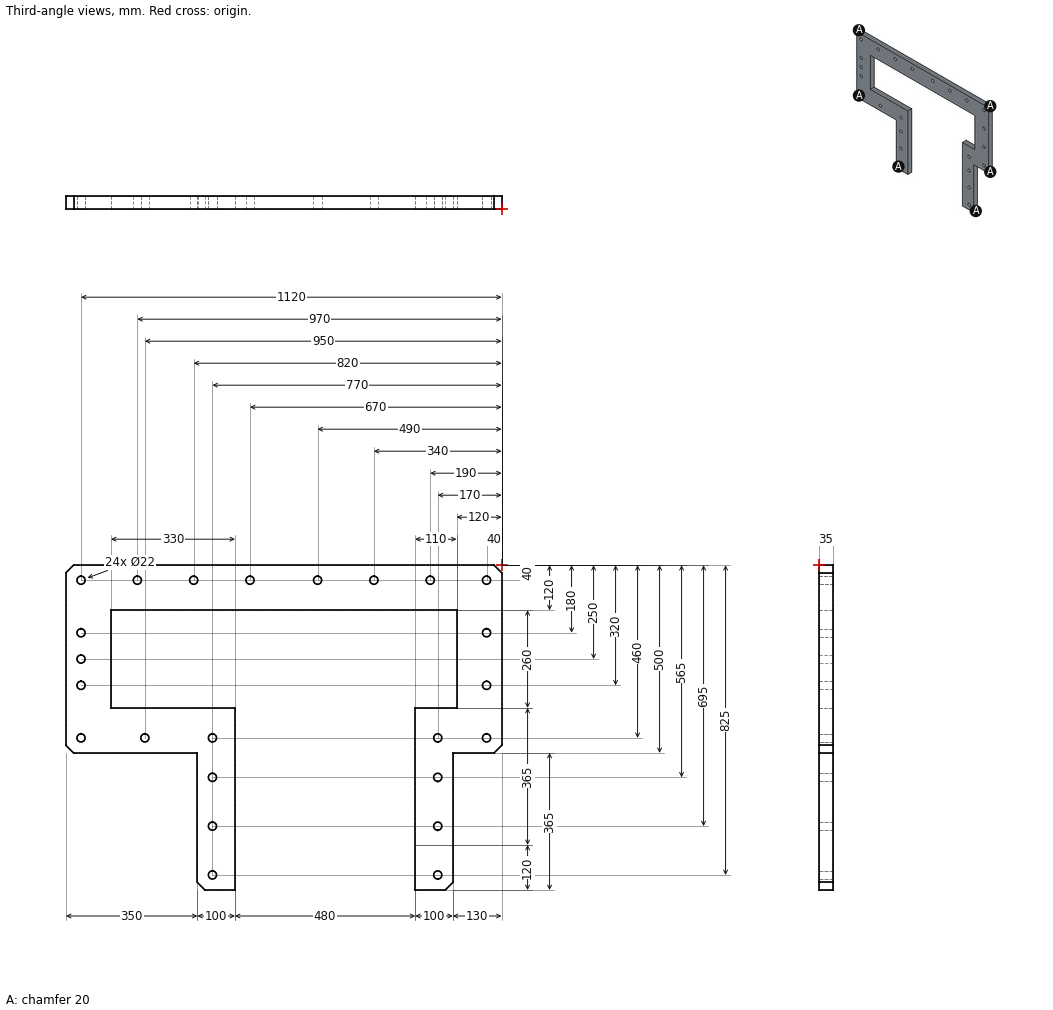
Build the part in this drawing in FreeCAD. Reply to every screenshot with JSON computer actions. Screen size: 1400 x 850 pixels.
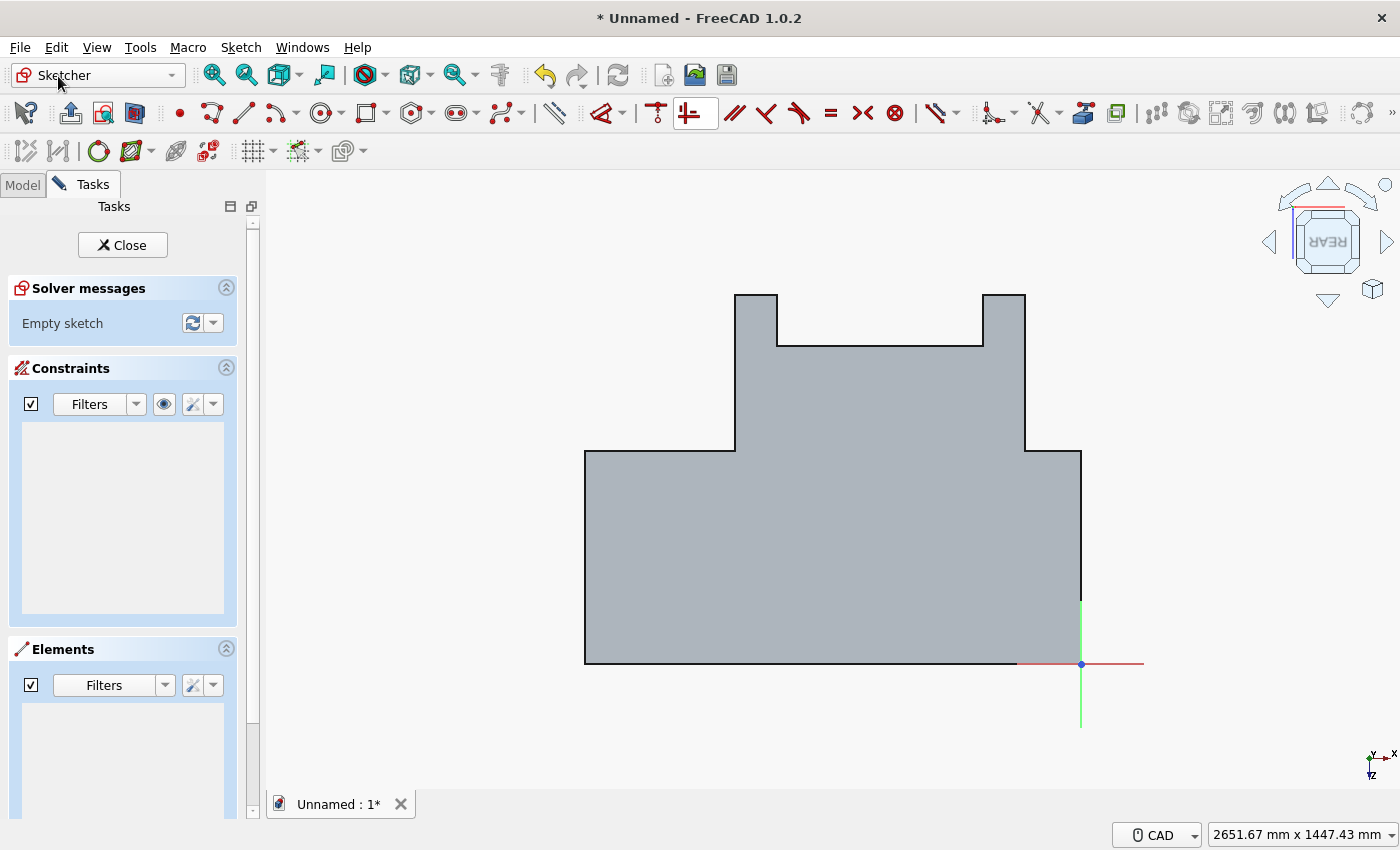
{"action": "key", "text": "g m"}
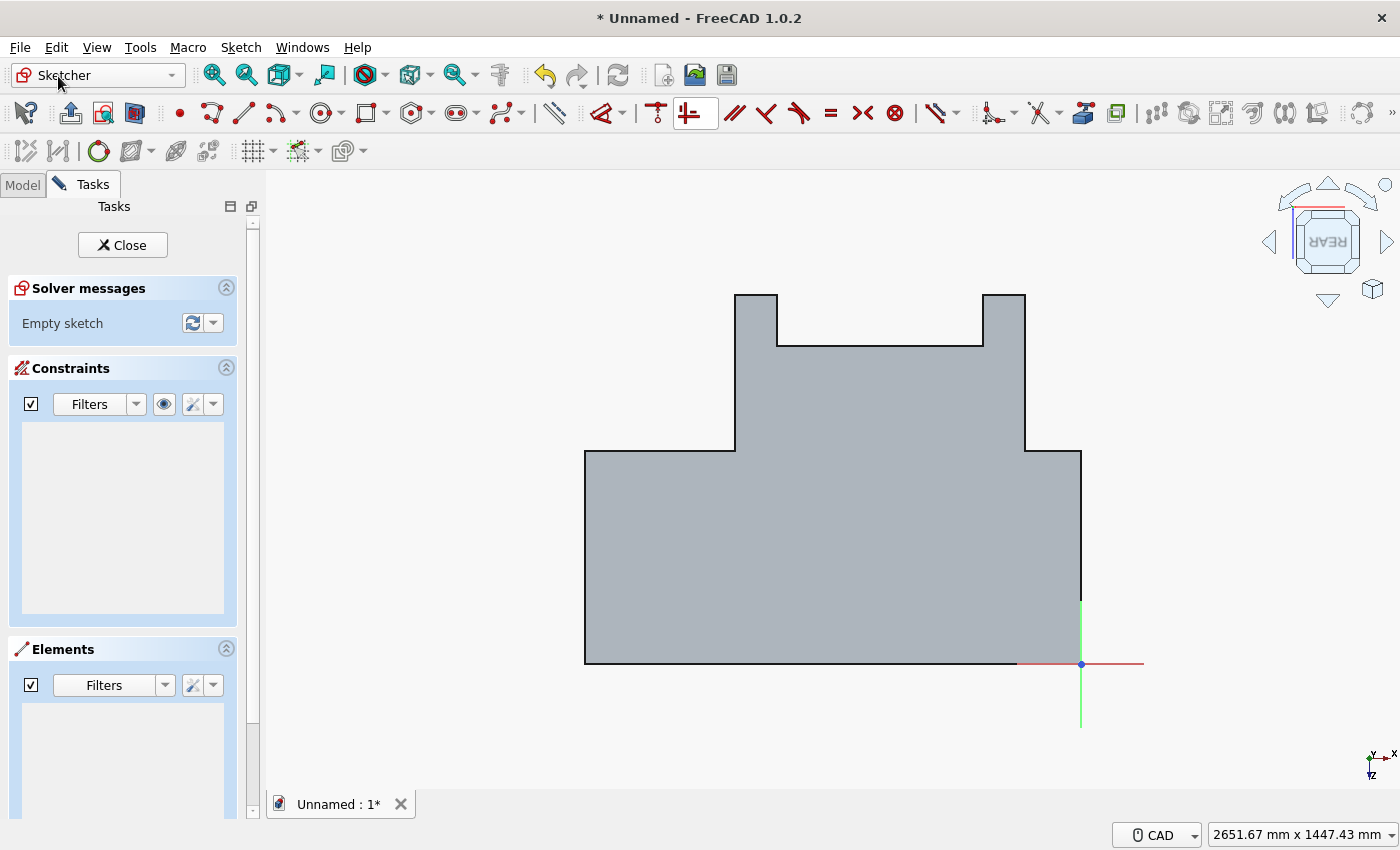
{"action": "left_click", "coordinate": [1030, 613]}
{"action": "left_click", "coordinate": [1030, 502]}
{"action": "left_click", "coordinate": [983, 502]}
{"action": "left_click", "coordinate": [983, 346]}
{"action": "left_click", "coordinate": [777, 346]}
{"action": "left_click", "coordinate": [777, 502]}
{"action": "left_click", "coordinate": [636, 502]}
{"action": "left_click", "coordinate": [636, 613]}
{"action": "left_click", "coordinate": [1030, 614]}
{"action": "key", "text": "Escape"}
{"action": "key", "text": "Escape"}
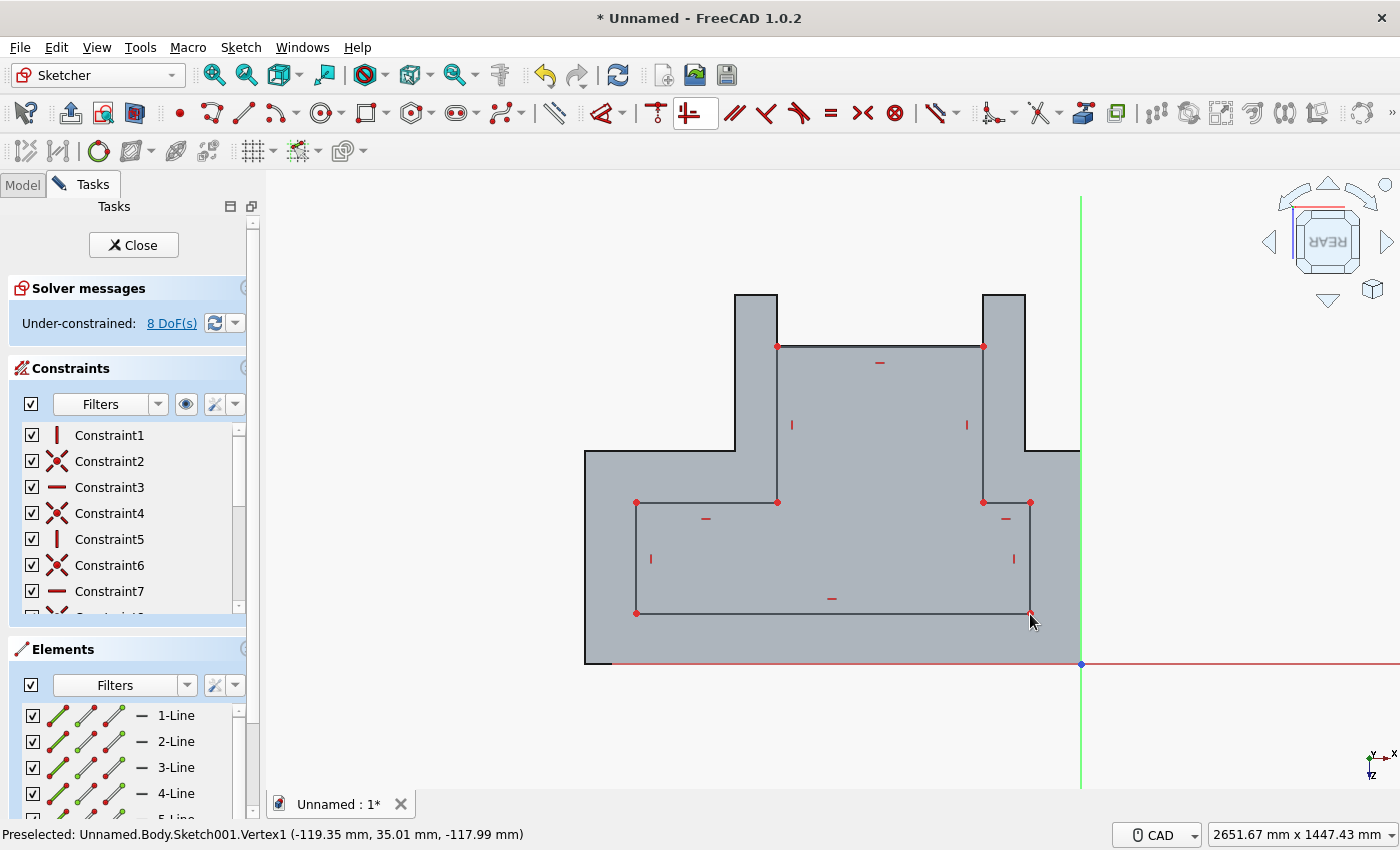
{"action": "key", "text": "d"}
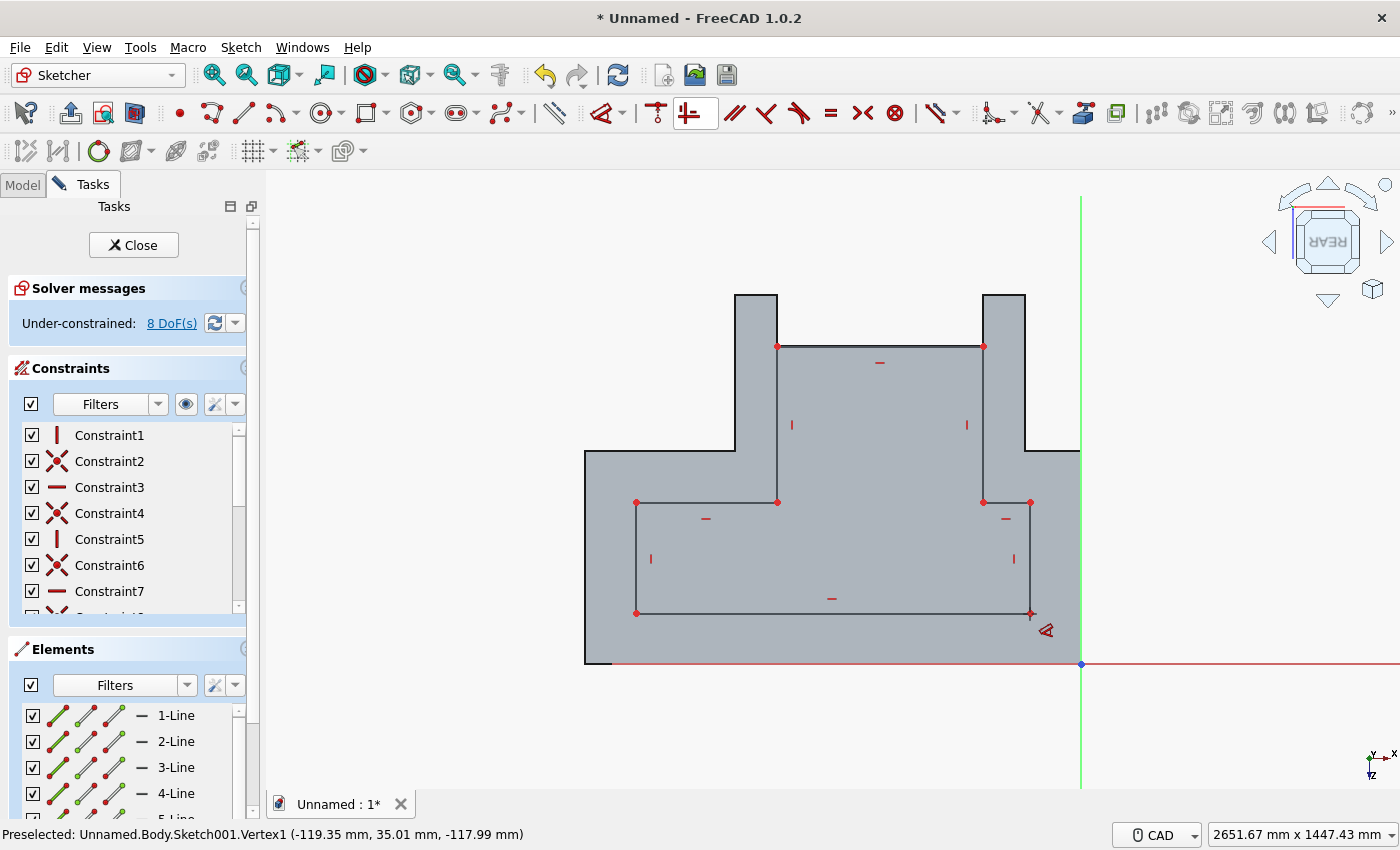
{"action": "left_click", "coordinate": [1030, 581]}
{"action": "left_click", "coordinate": [1064, 558]}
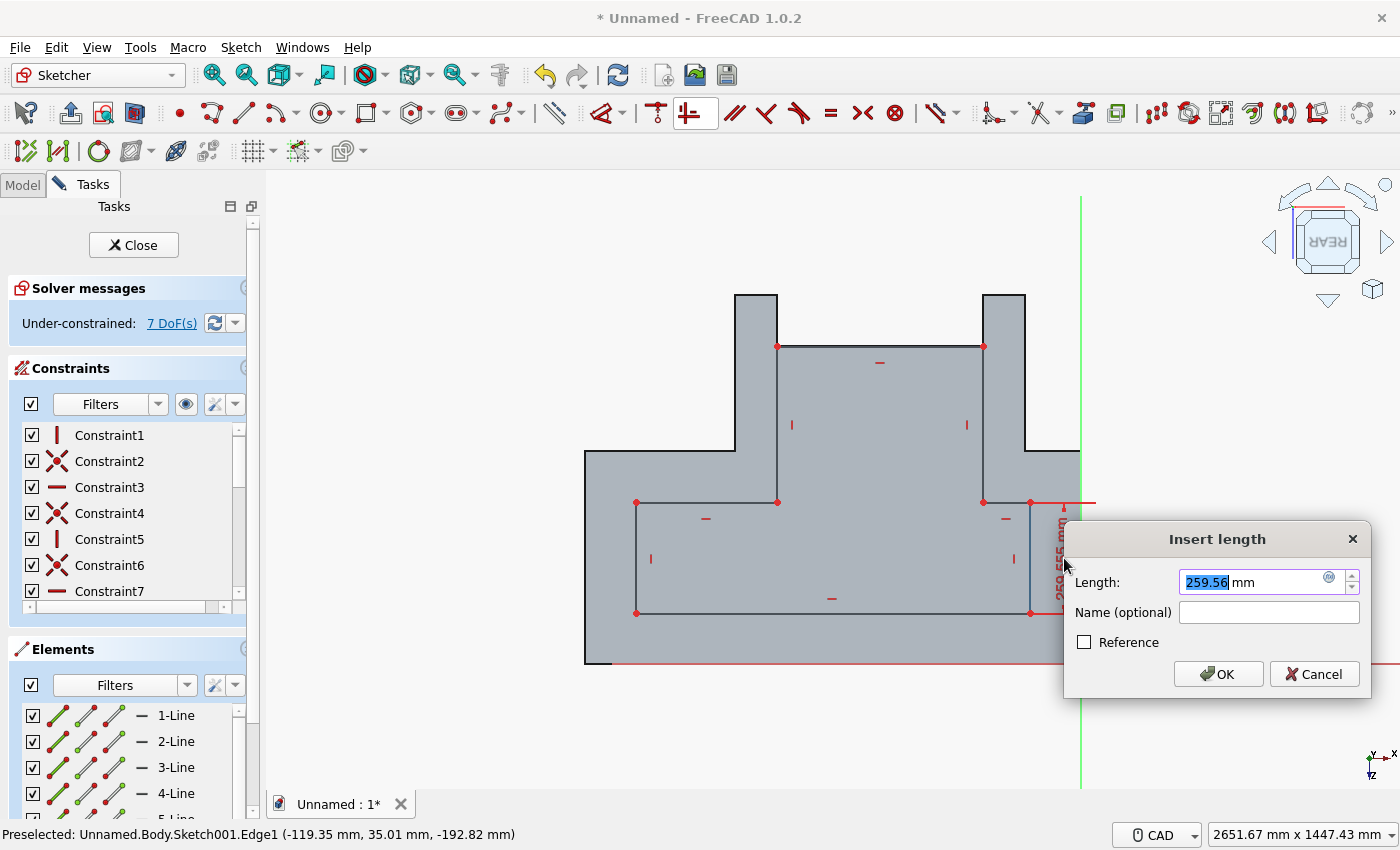
{"action": "type", "text": "260"}
{"action": "key", "text": "Return"}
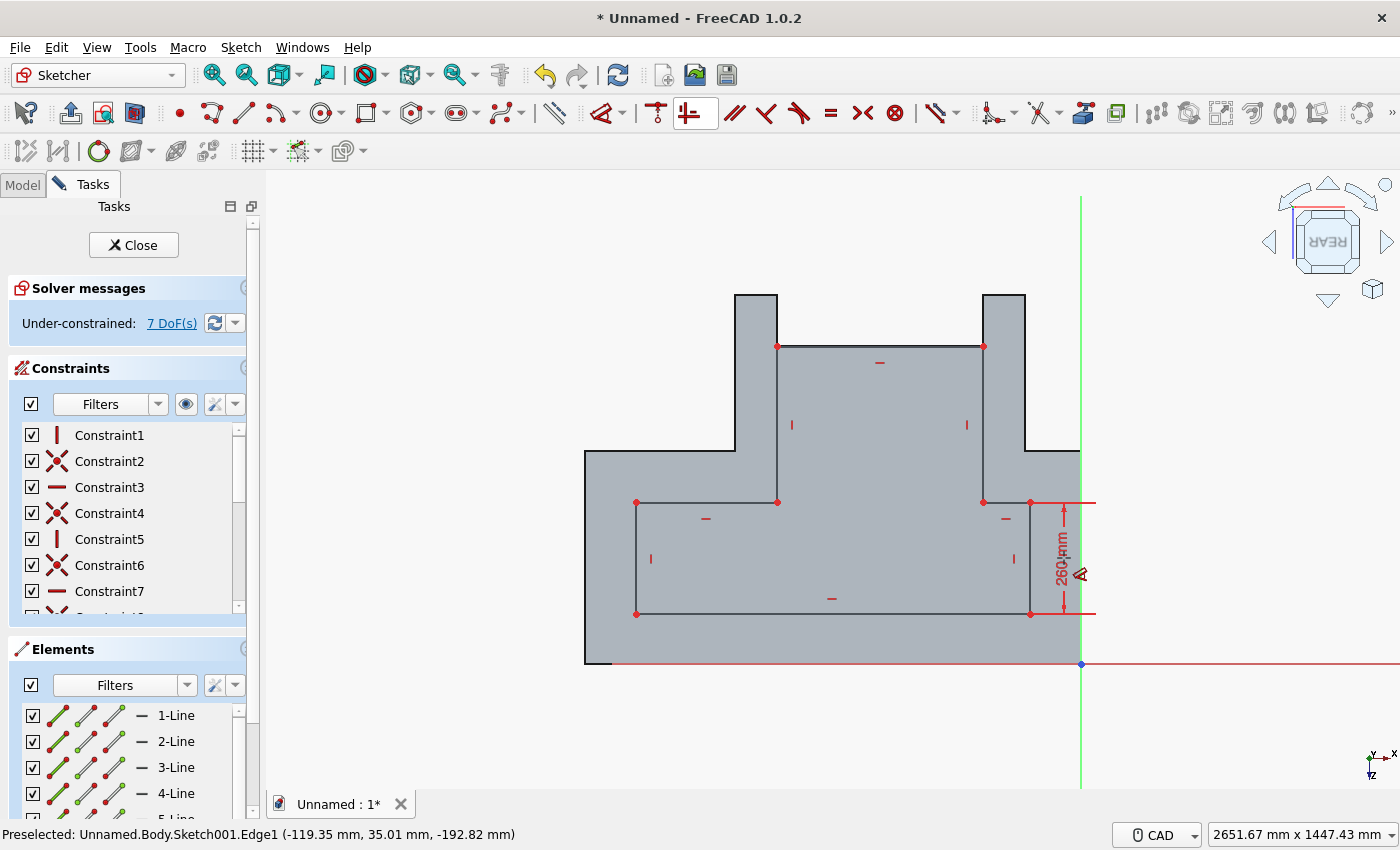
{"action": "left_click", "coordinate": [1016, 503]}
{"action": "left_click", "coordinate": [1006, 469]}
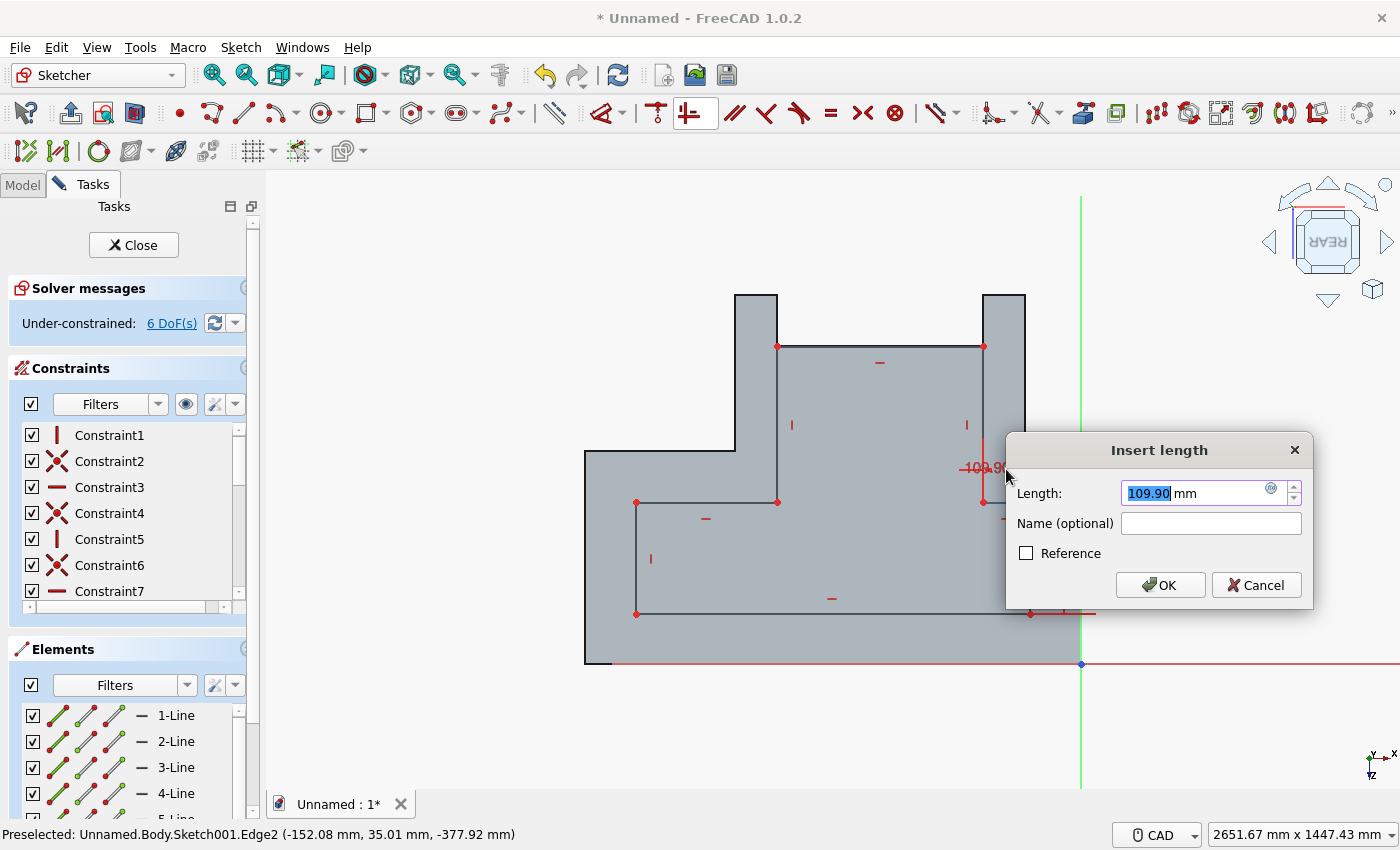
{"action": "type", "text": "110"}
{"action": "key", "text": "Return"}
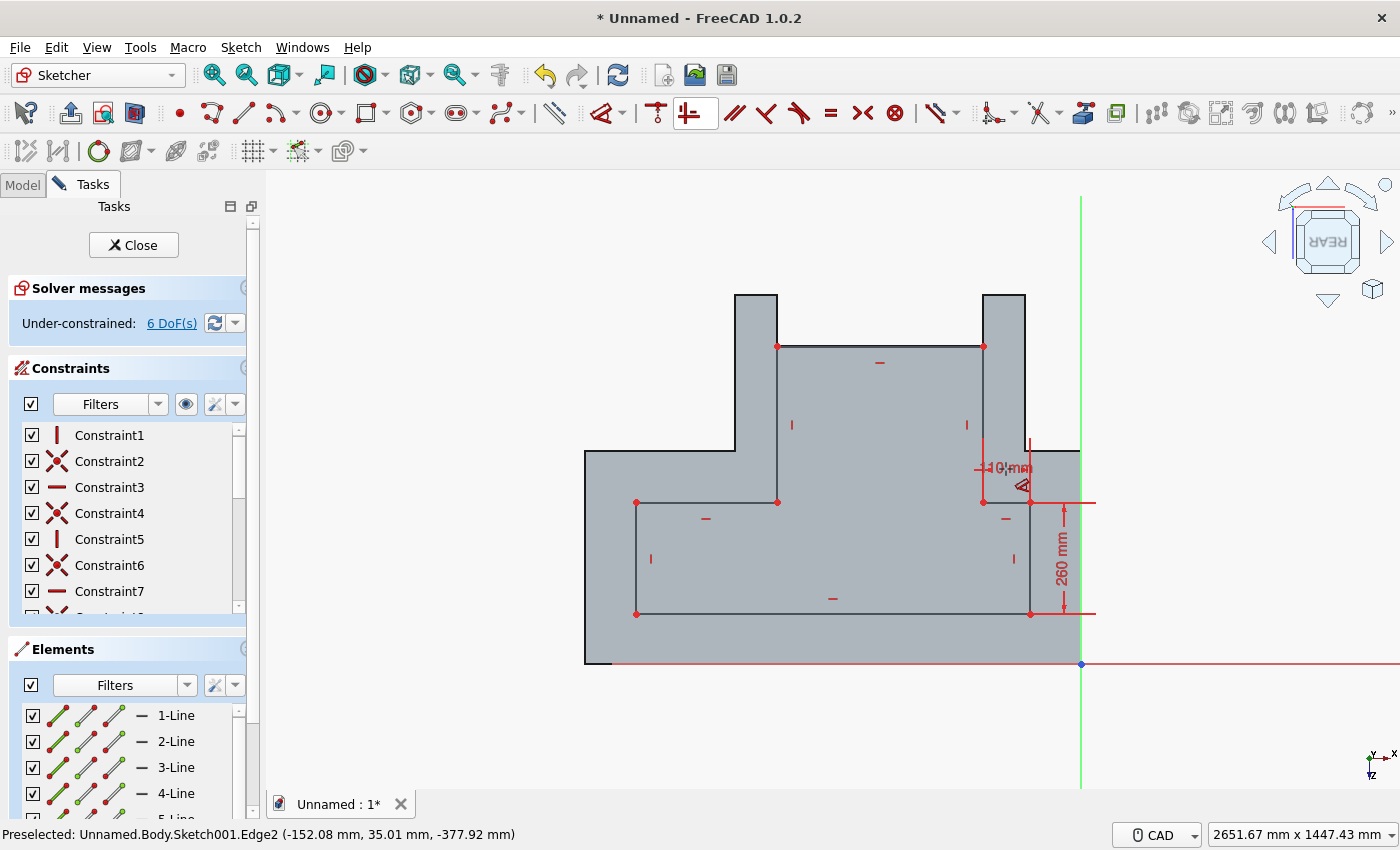
{"action": "left_click", "coordinate": [983, 456]}
{"action": "left_click", "coordinate": [1017, 425]}